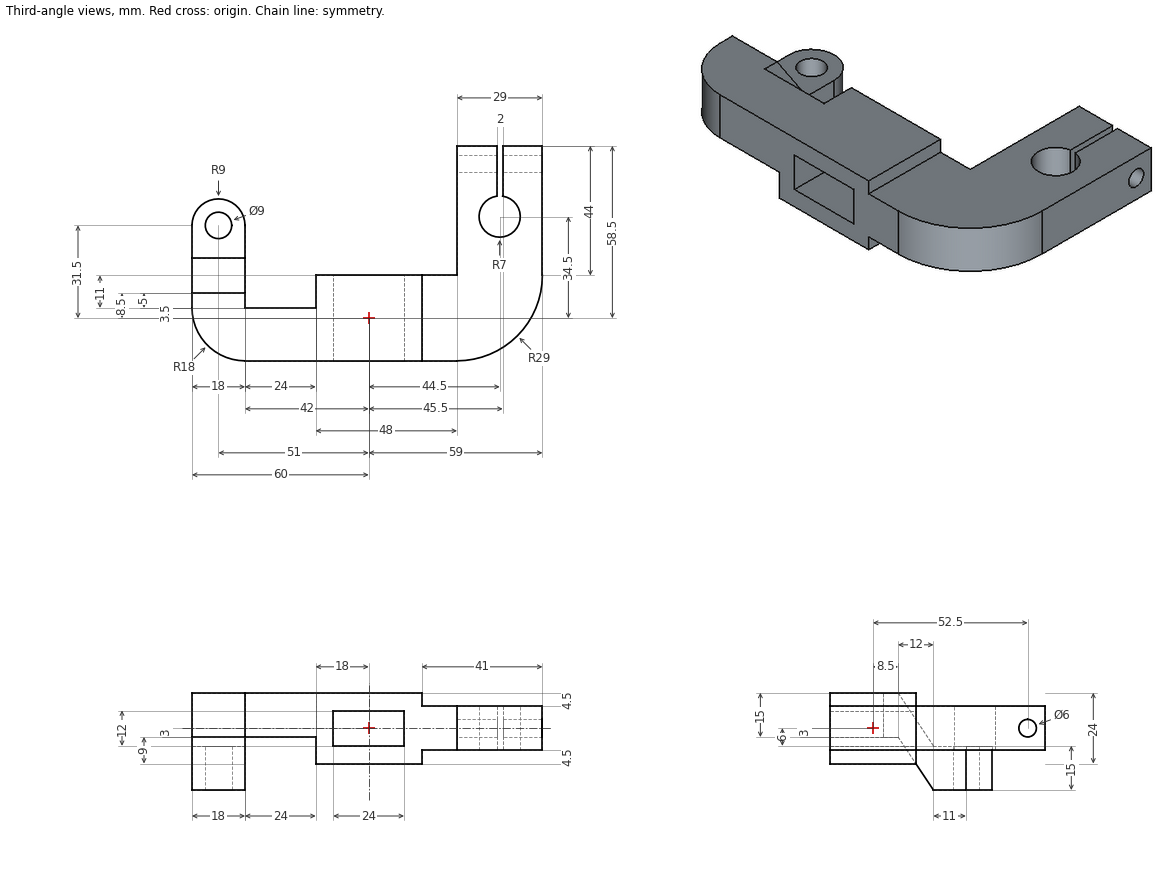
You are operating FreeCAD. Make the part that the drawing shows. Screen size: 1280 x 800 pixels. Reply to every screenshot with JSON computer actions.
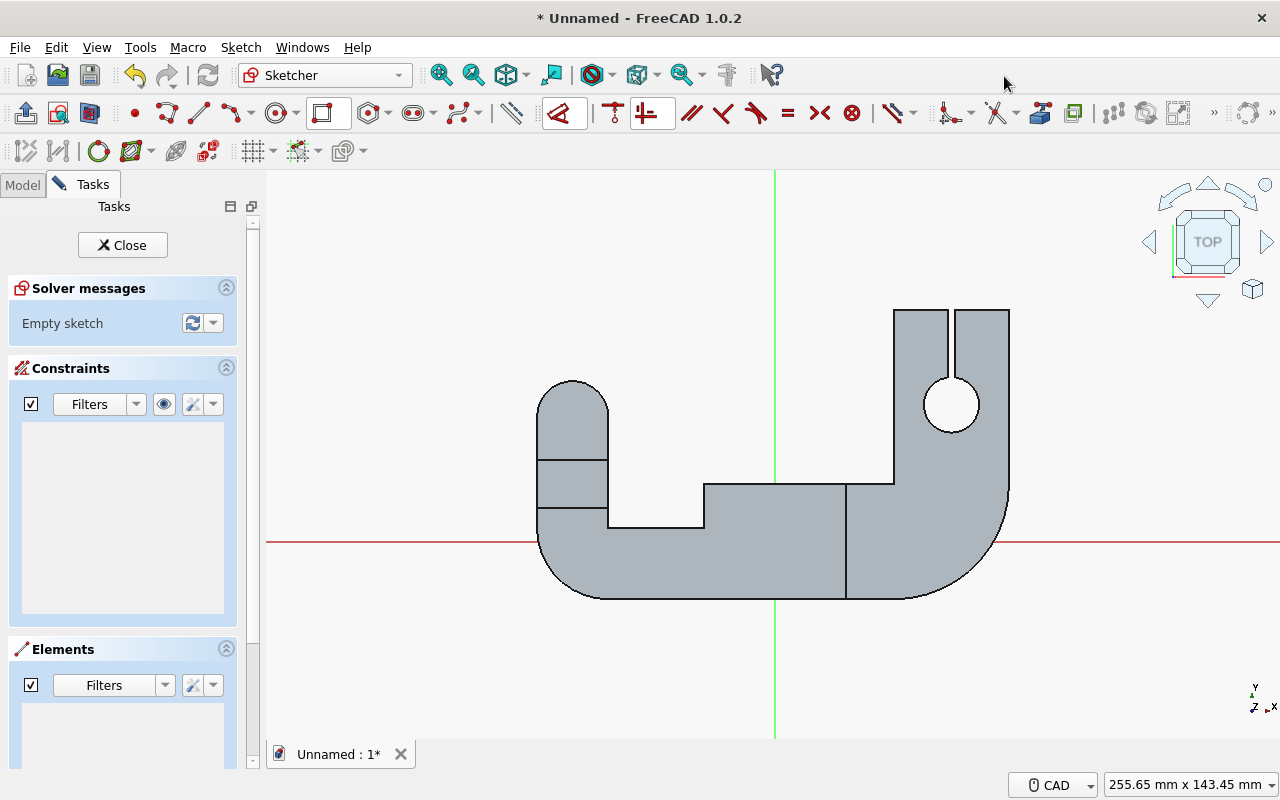
{"action": "scroll", "coordinate": [560, 413], "scroll_direction": "up", "scroll_amount": 12}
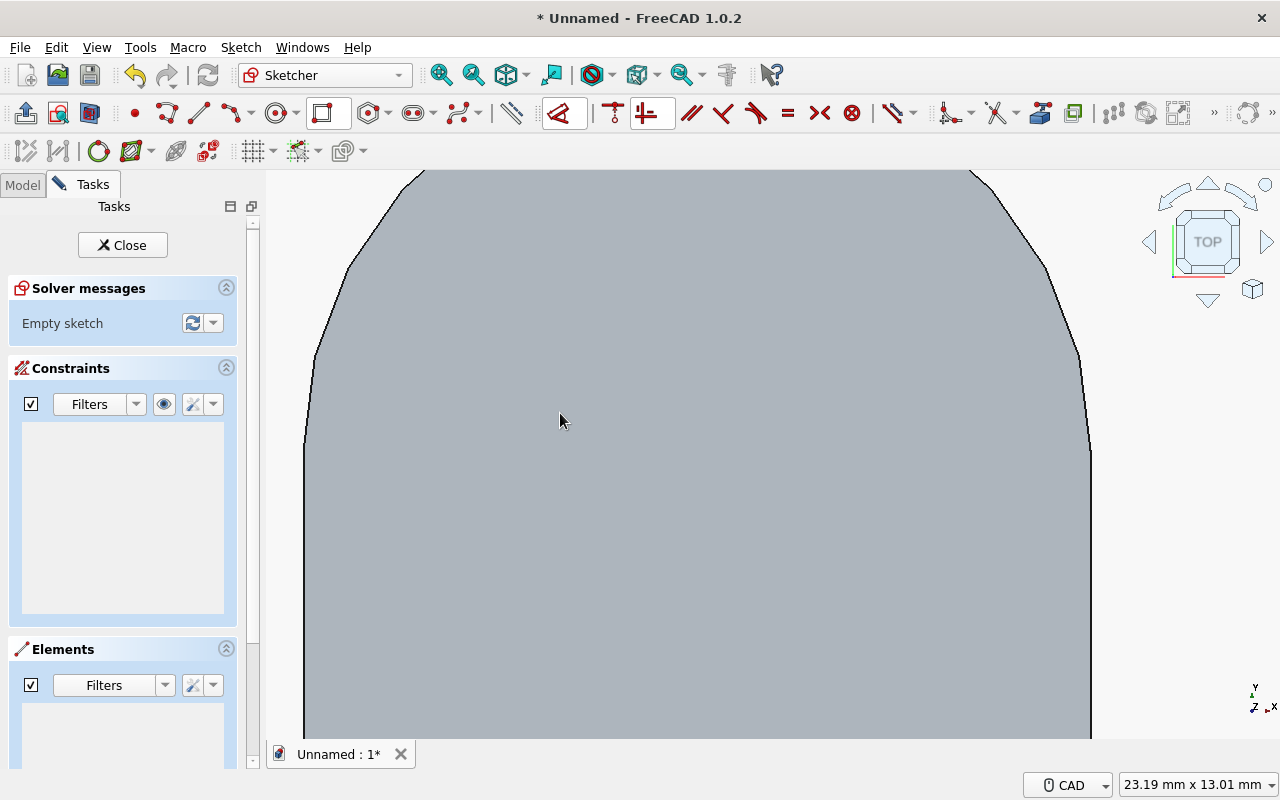
{"action": "left_click", "coordinate": [276, 114]}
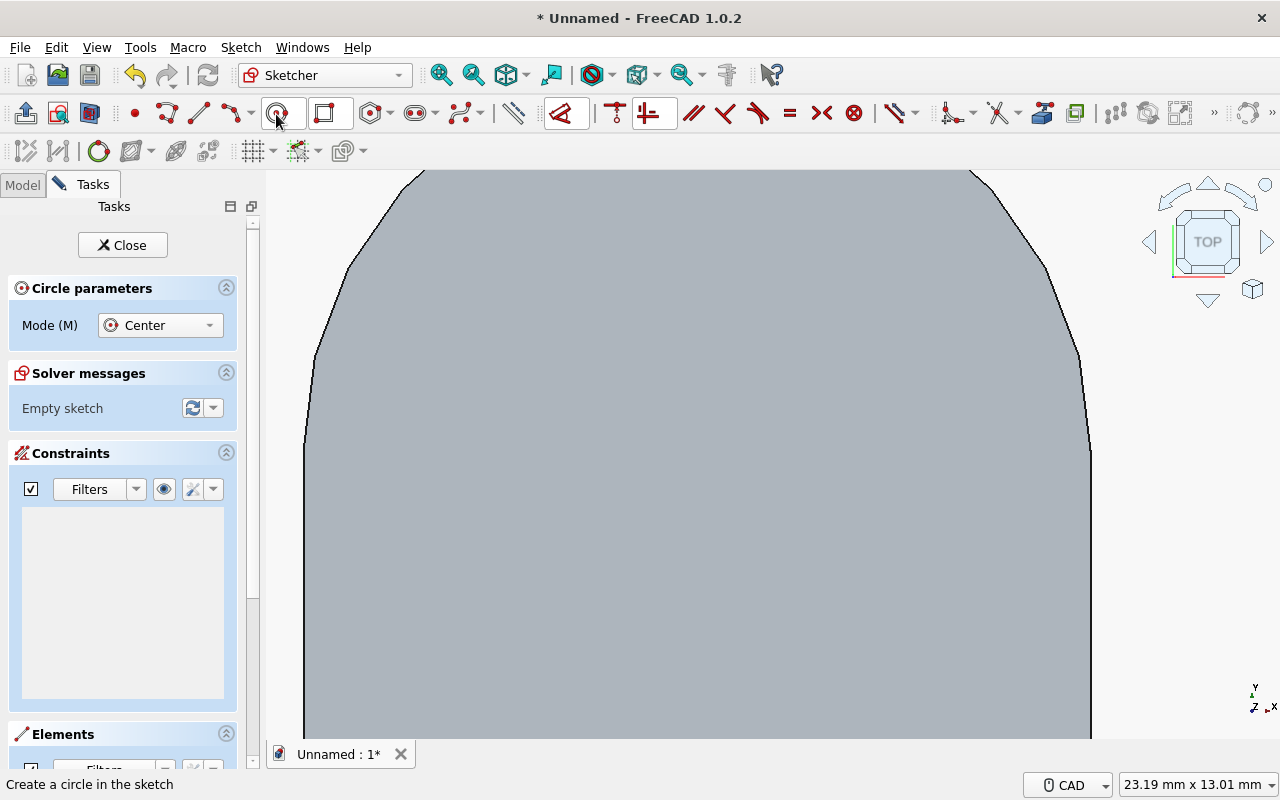
{"action": "left_click", "coordinate": [697, 451]}
{"action": "mouse_move", "coordinate": [836, 312]}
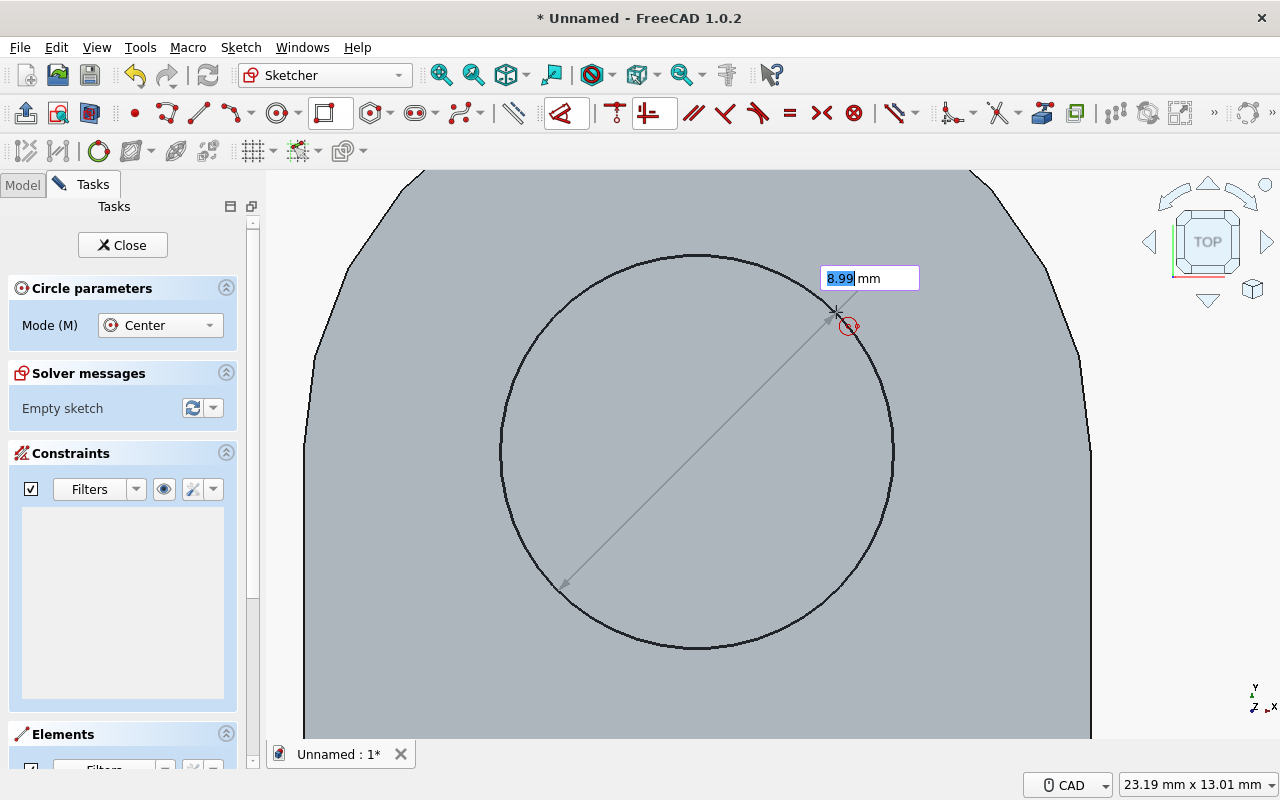
{"action": "type", "text": "9"}
{"action": "key", "text": "Return"}
{"action": "key", "text": "Escape"}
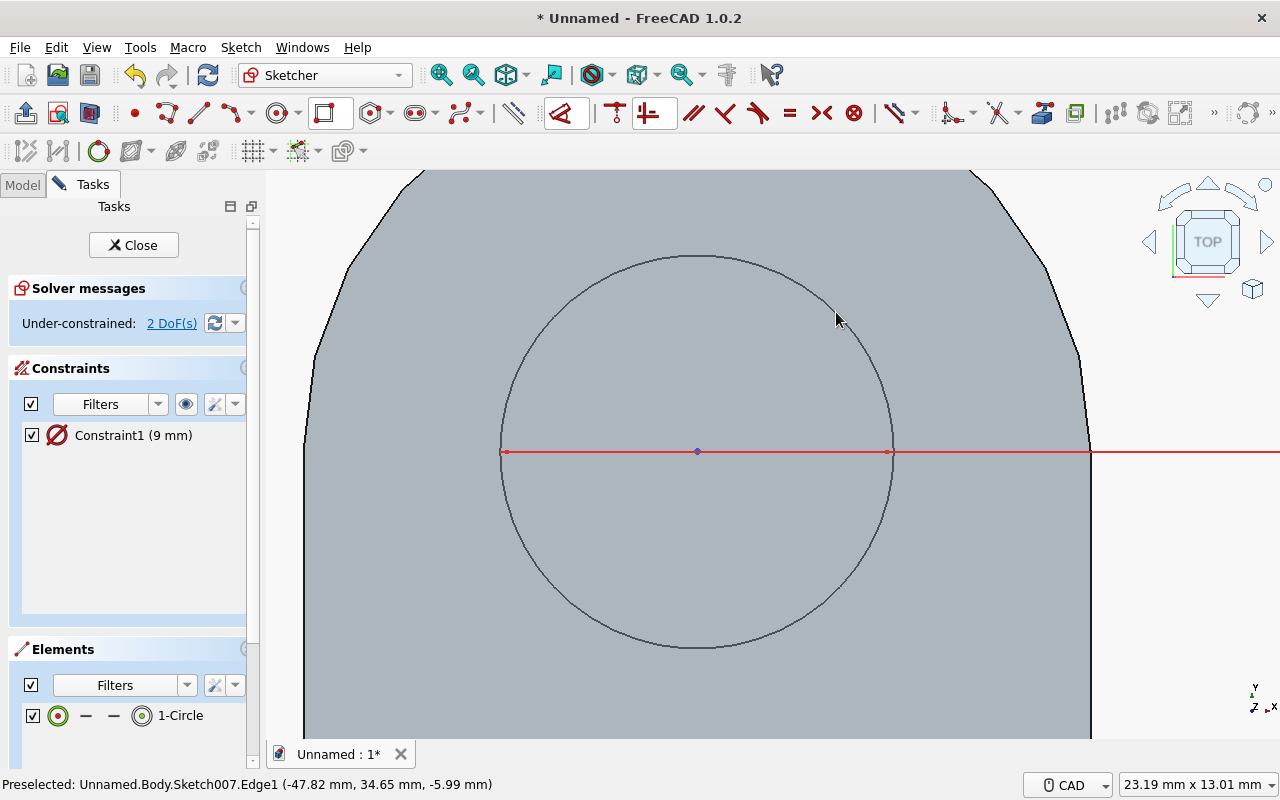
{"action": "left_click", "coordinate": [697, 452]}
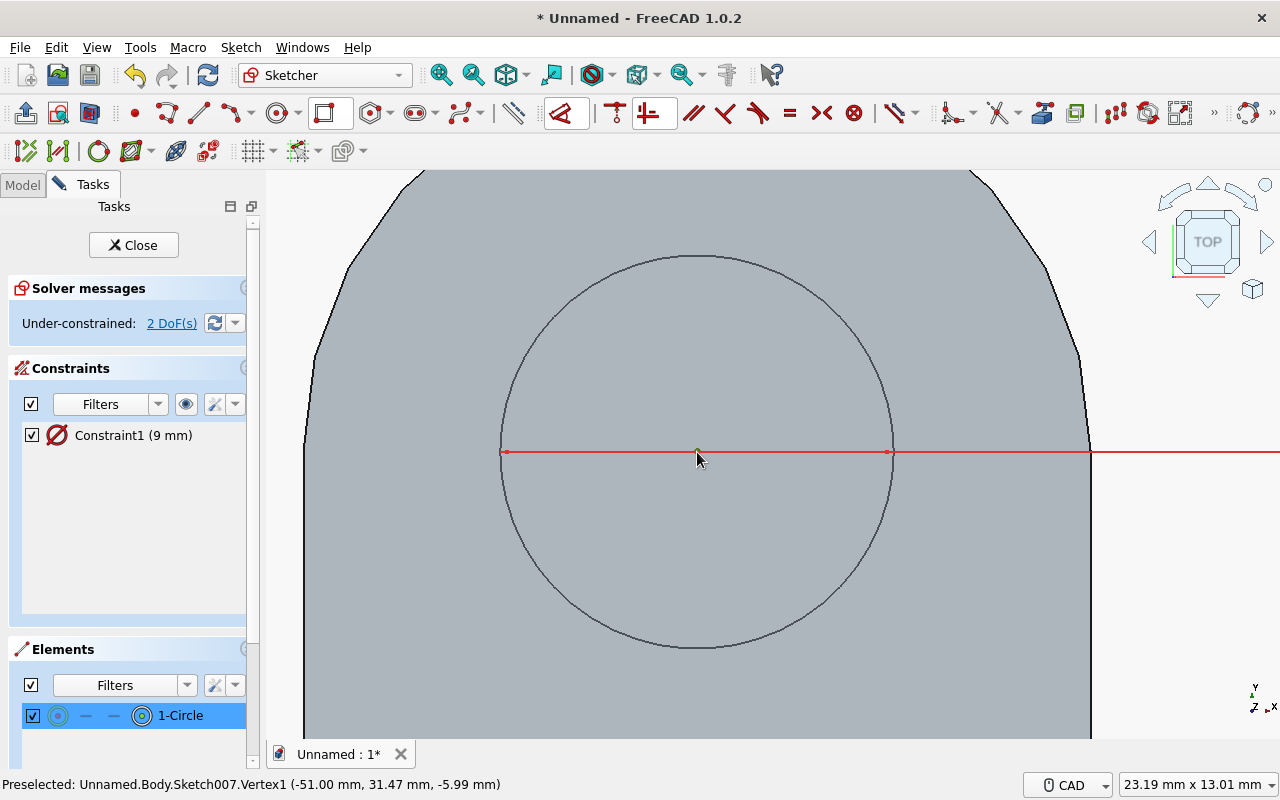
{"action": "left_click", "coordinate": [584, 114]}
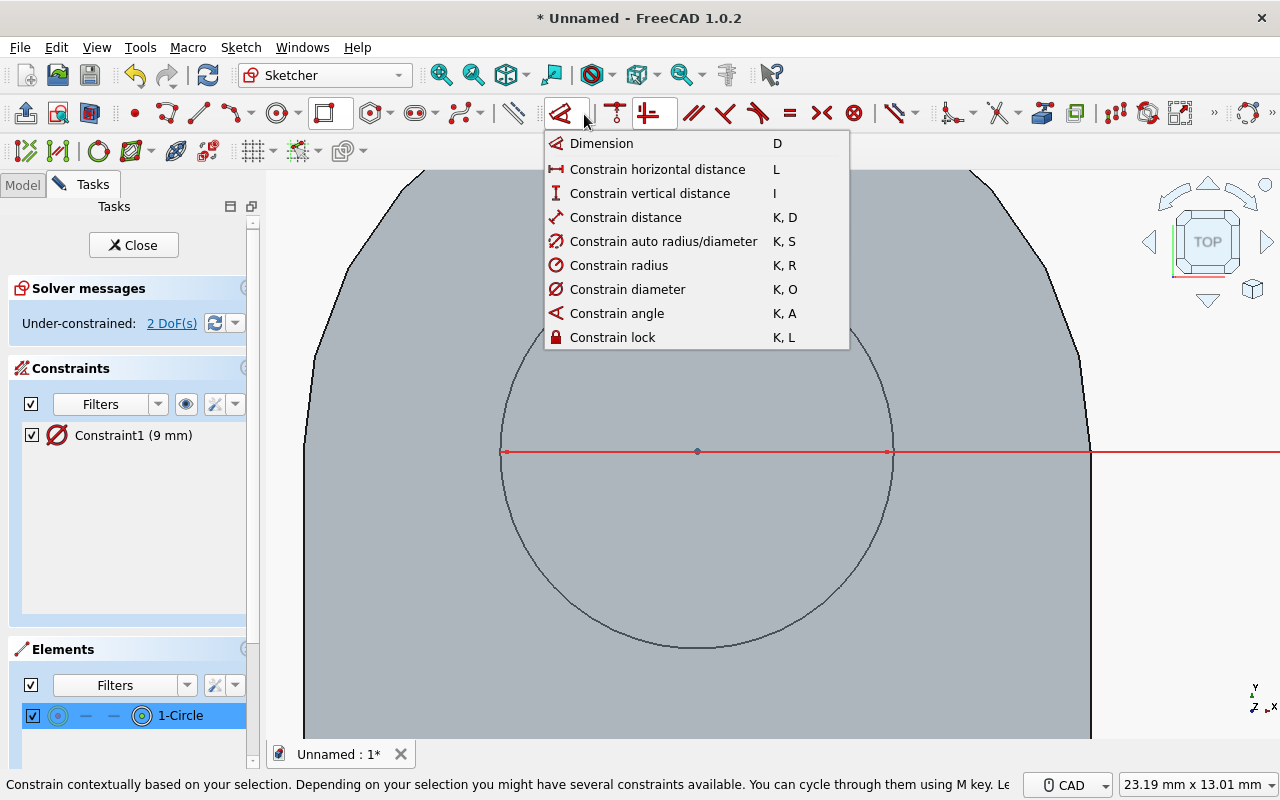
{"action": "left_click", "coordinate": [697, 169]}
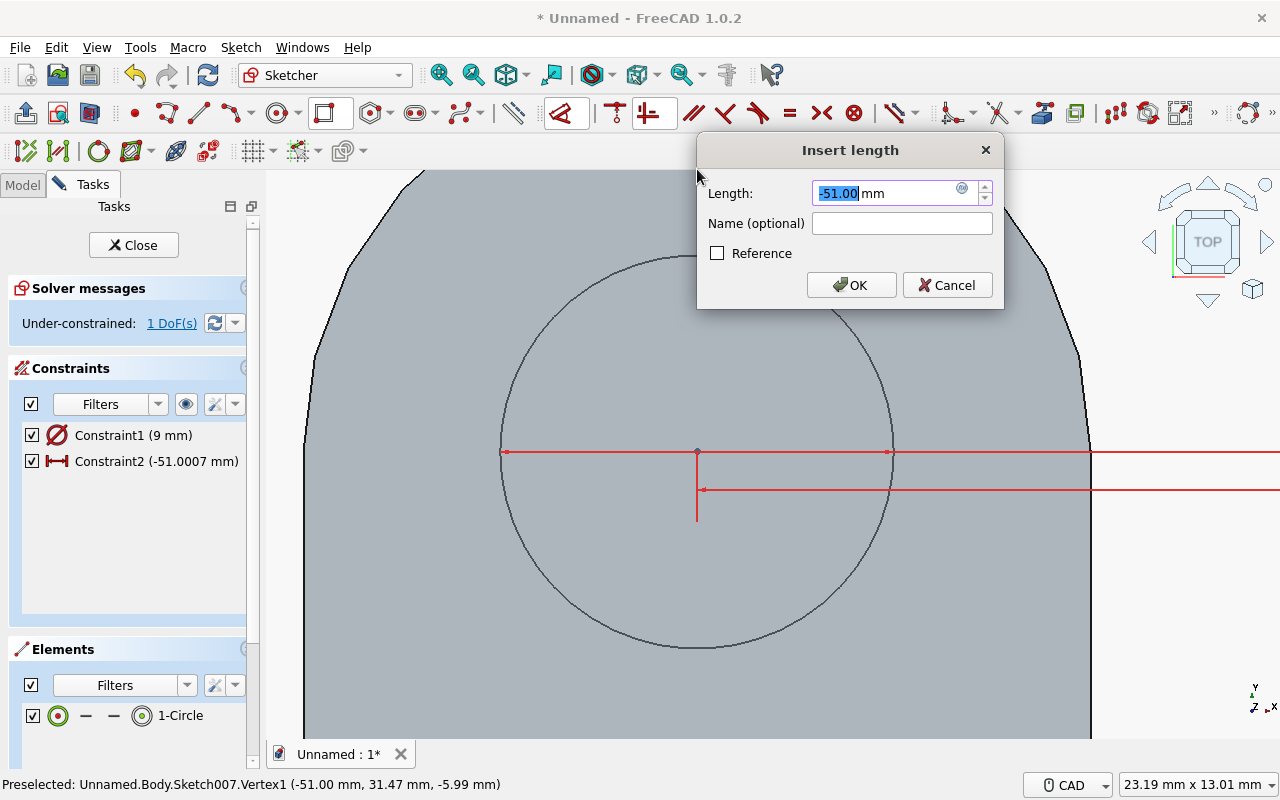
{"action": "type", "text": "-51"}
{"action": "key", "text": "Return"}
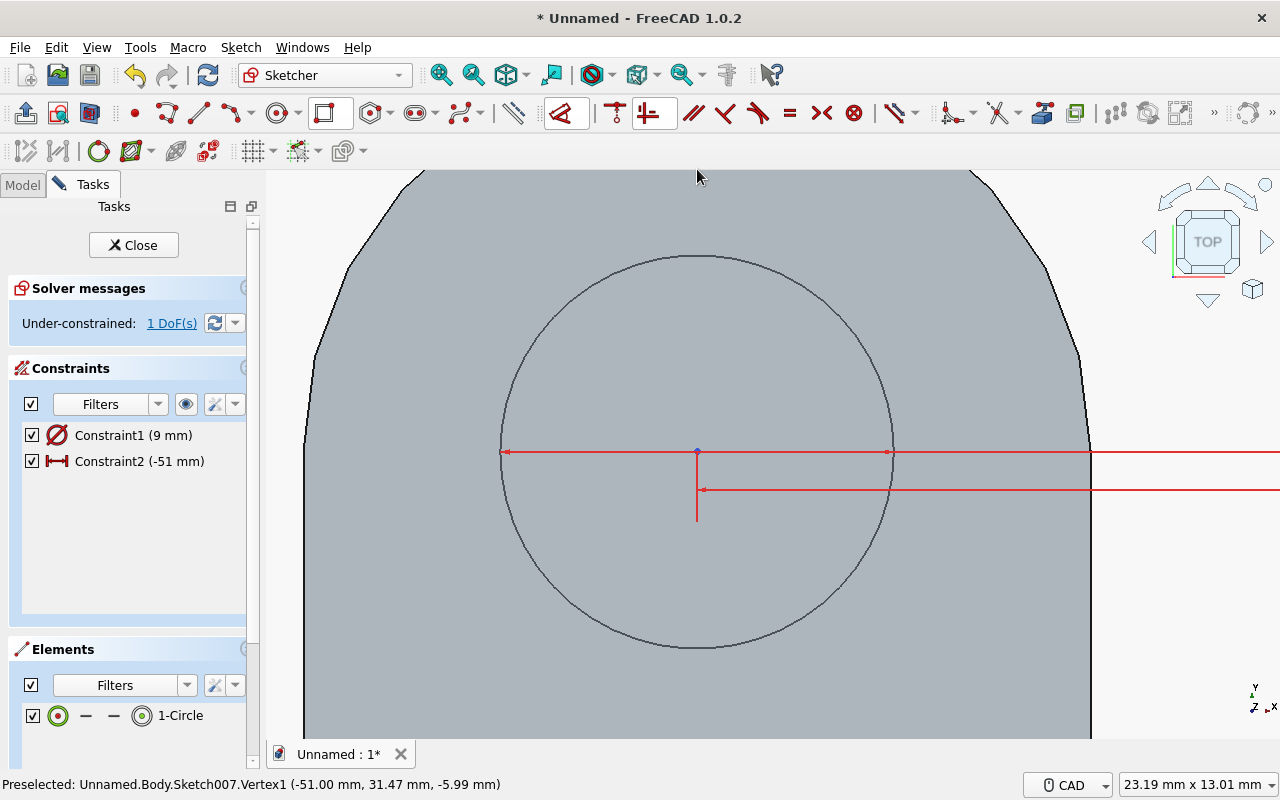
{"action": "left_click", "coordinate": [697, 452]}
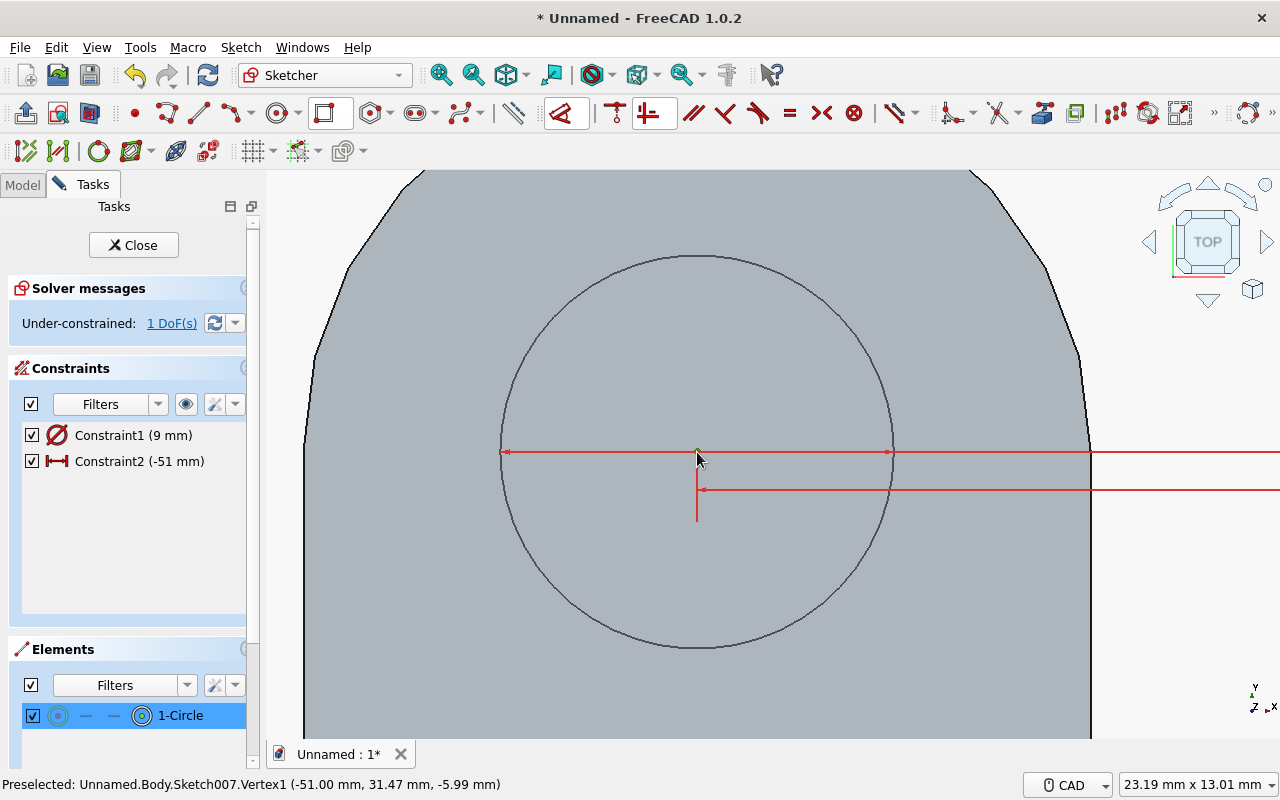
{"action": "key", "text": "i"}